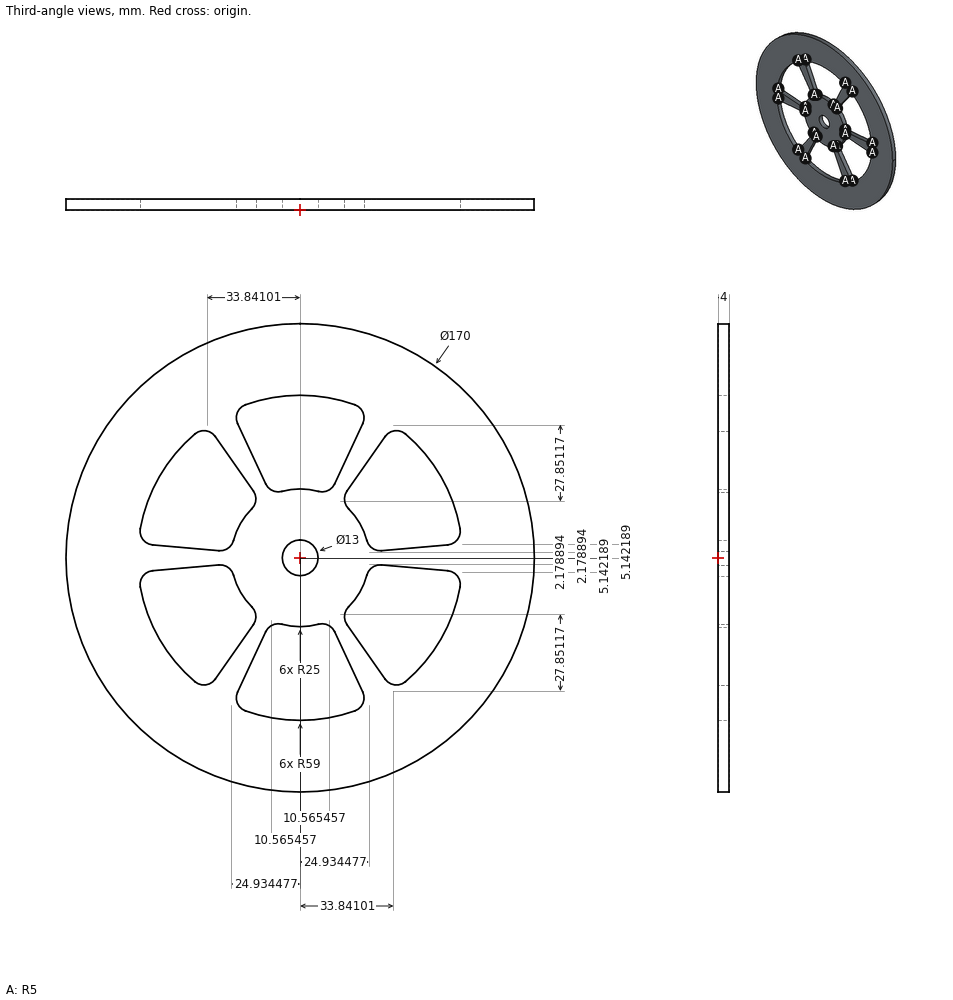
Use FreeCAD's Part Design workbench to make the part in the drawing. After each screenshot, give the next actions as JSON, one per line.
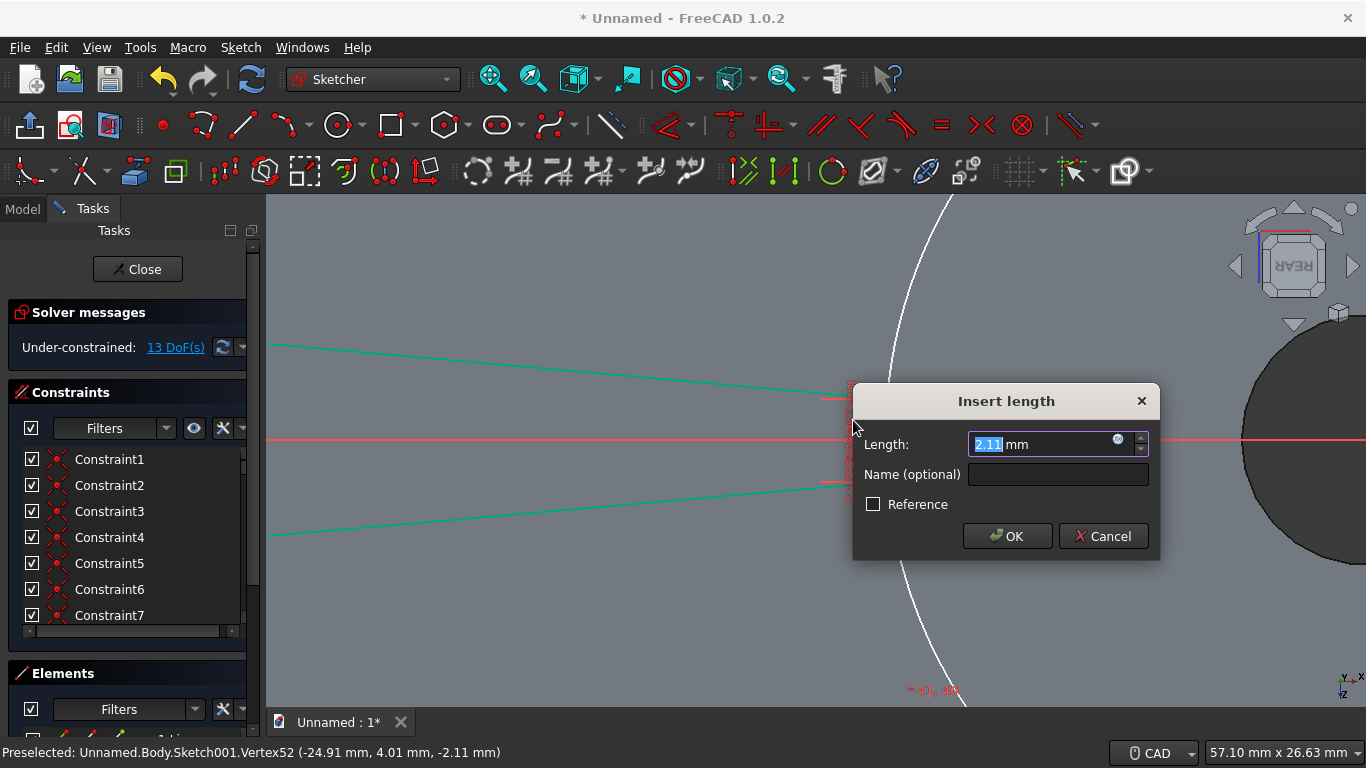
{"action": "type", "text": "2.178894"}
{"action": "key", "text": "Return"}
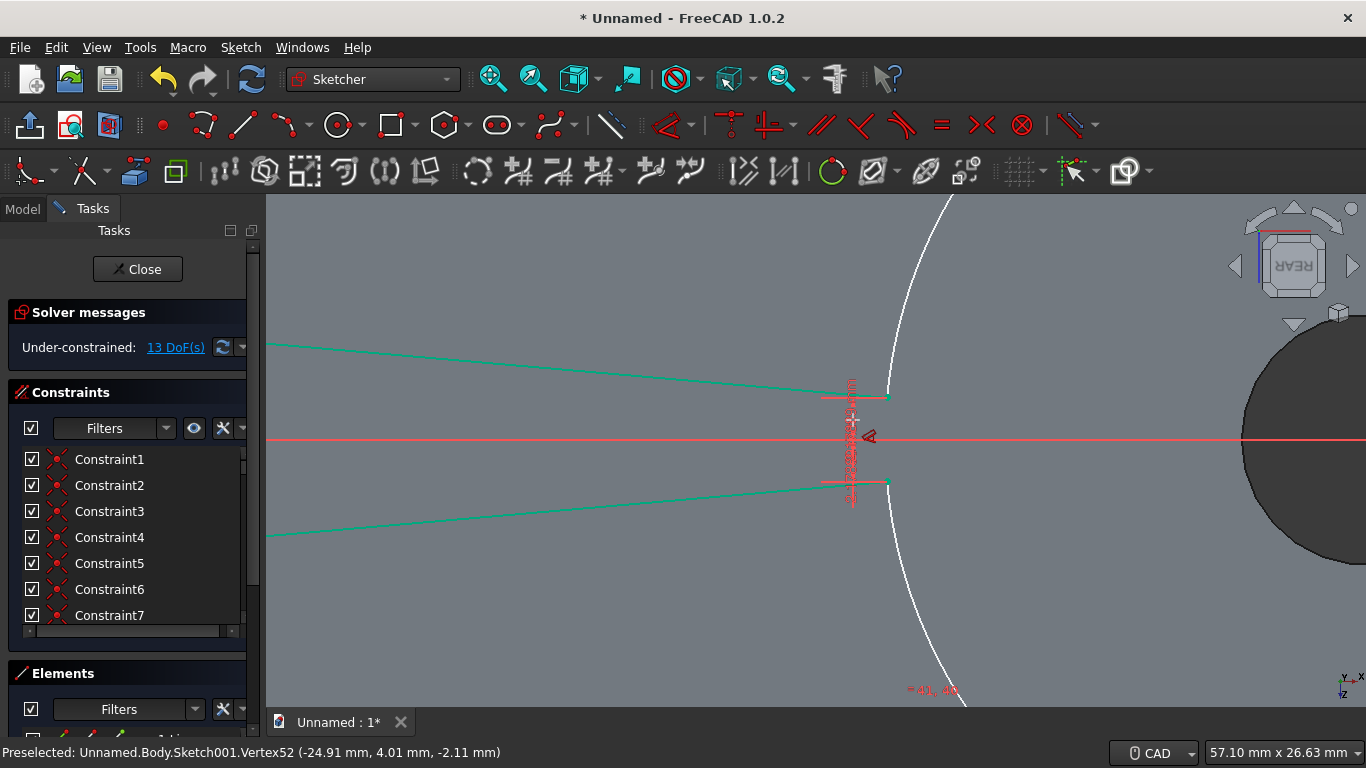
{"action": "scroll", "coordinate": [651, 452], "scroll_direction": "down", "scroll_amount": 10}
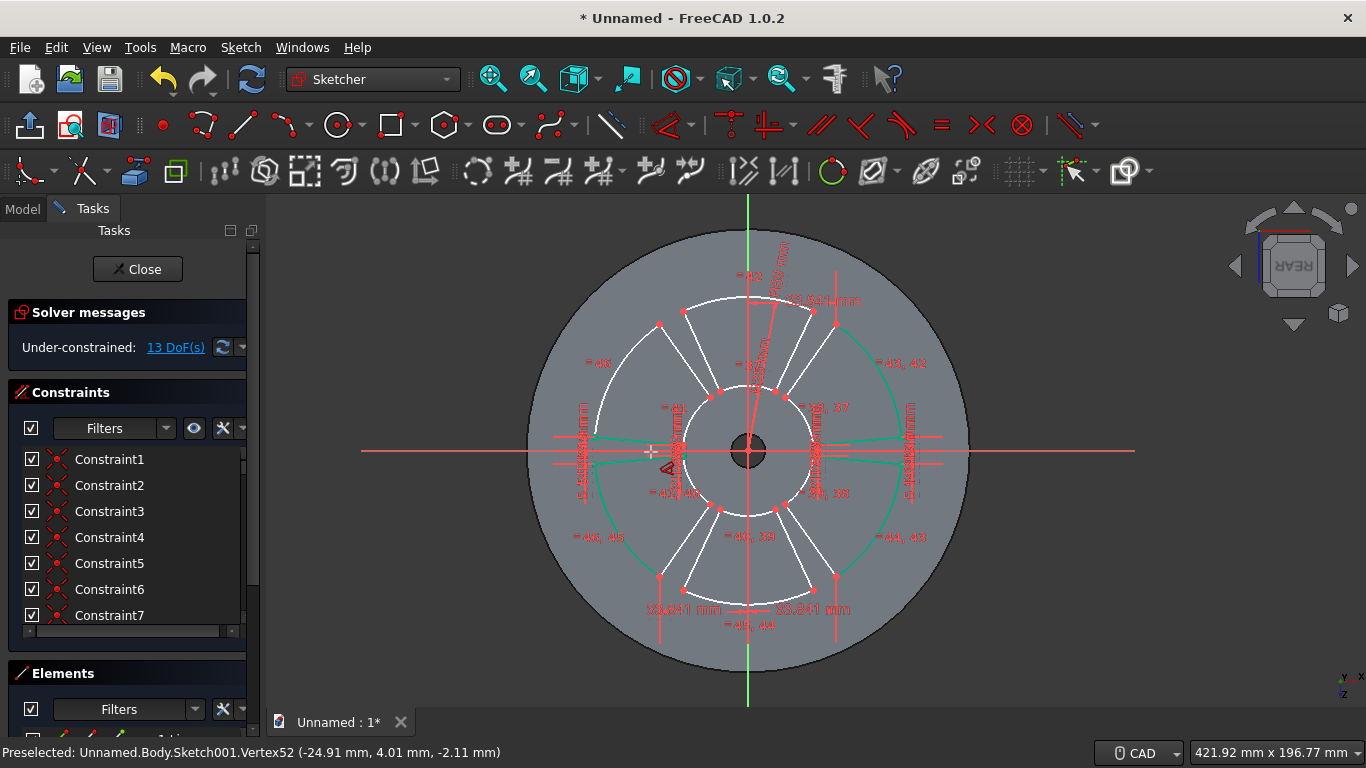
{"action": "left_click", "coordinate": [660, 325]}
{"action": "left_click", "coordinate": [684, 291]}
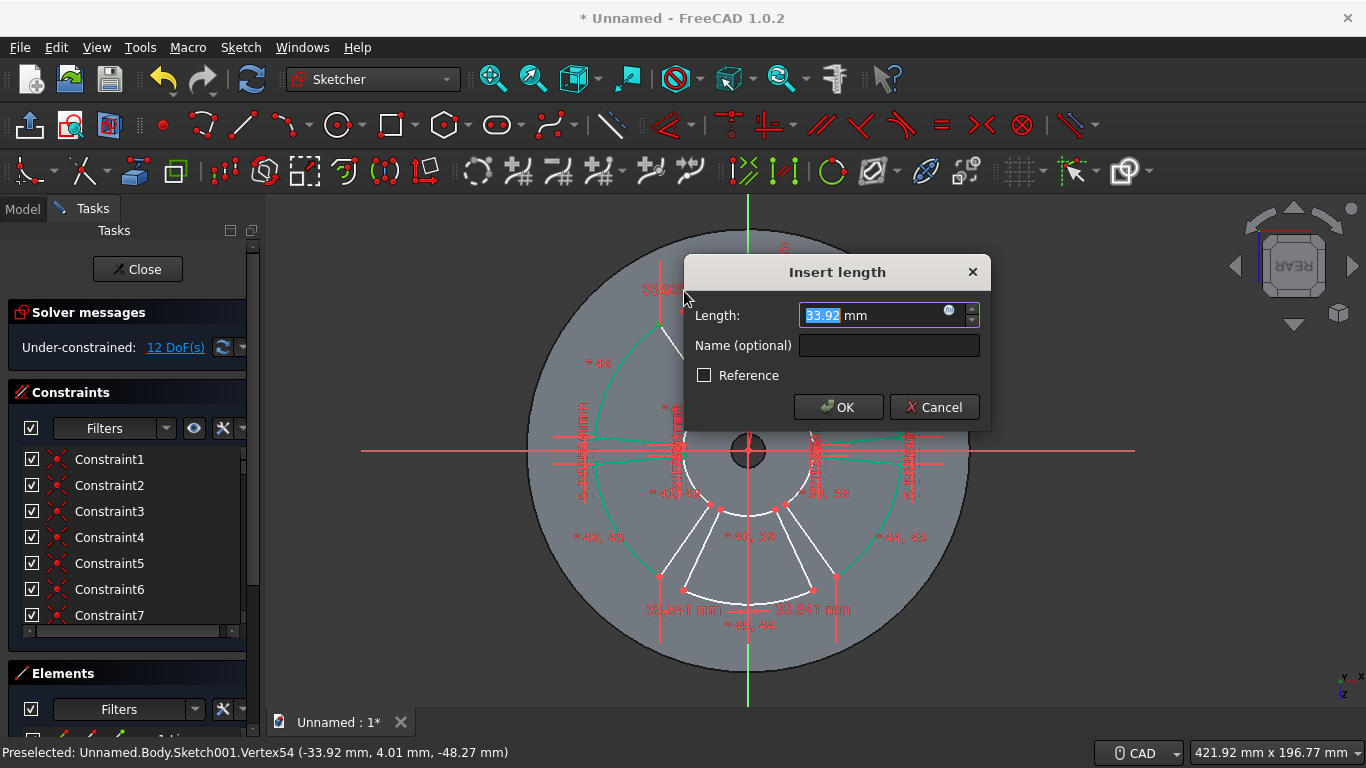
{"action": "type", "text": "33.84101"}
{"action": "key", "text": "Return"}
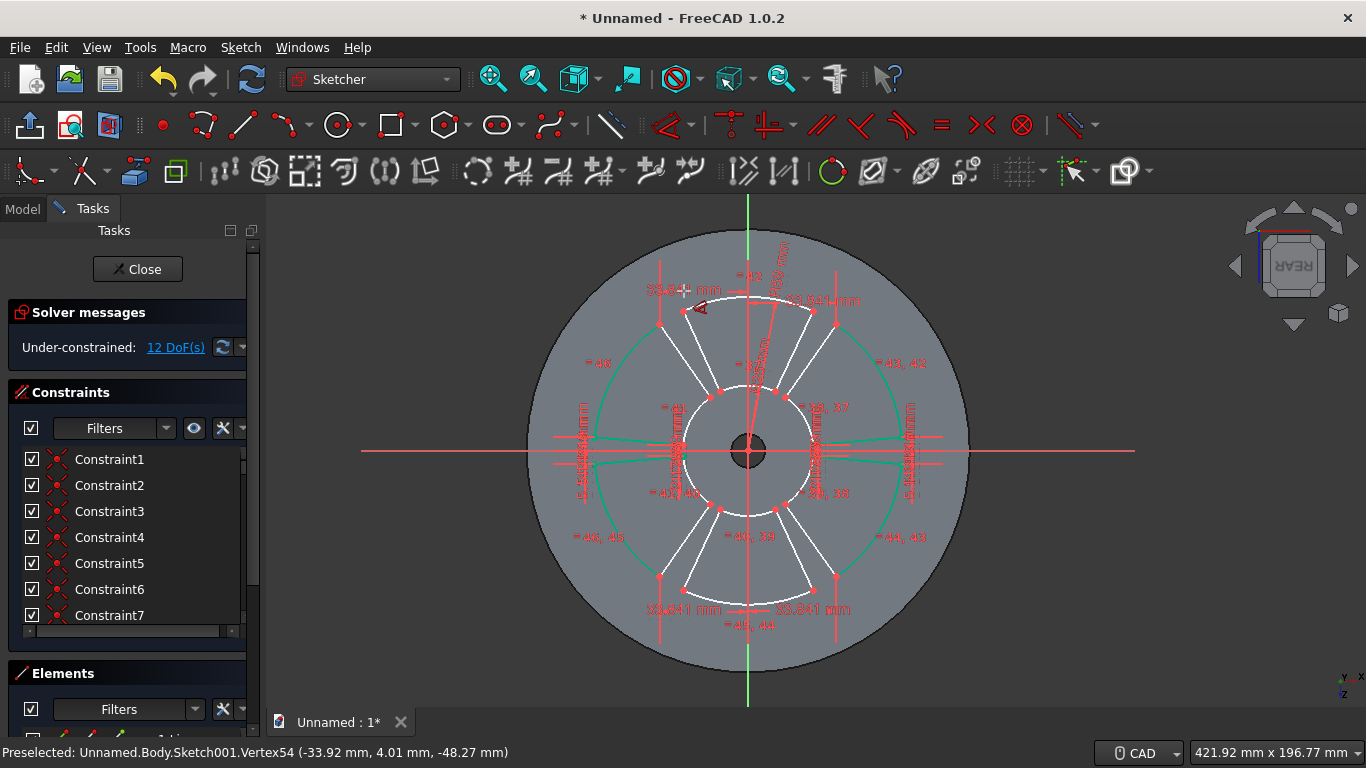
{"action": "left_click", "coordinate": [821, 347]}
{"action": "left_click", "coordinate": [870, 336]}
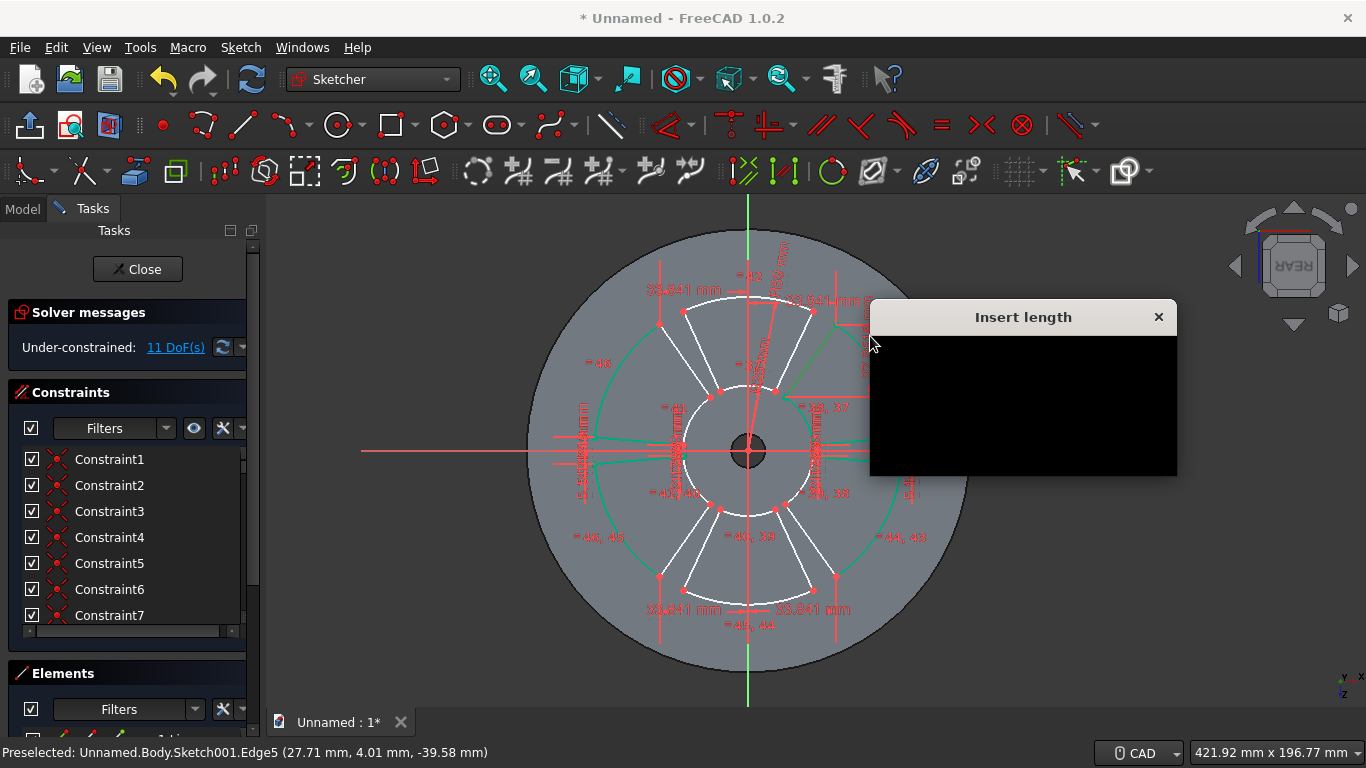
{"action": "type", "text": "27.85117"}
{"action": "key", "text": "Return"}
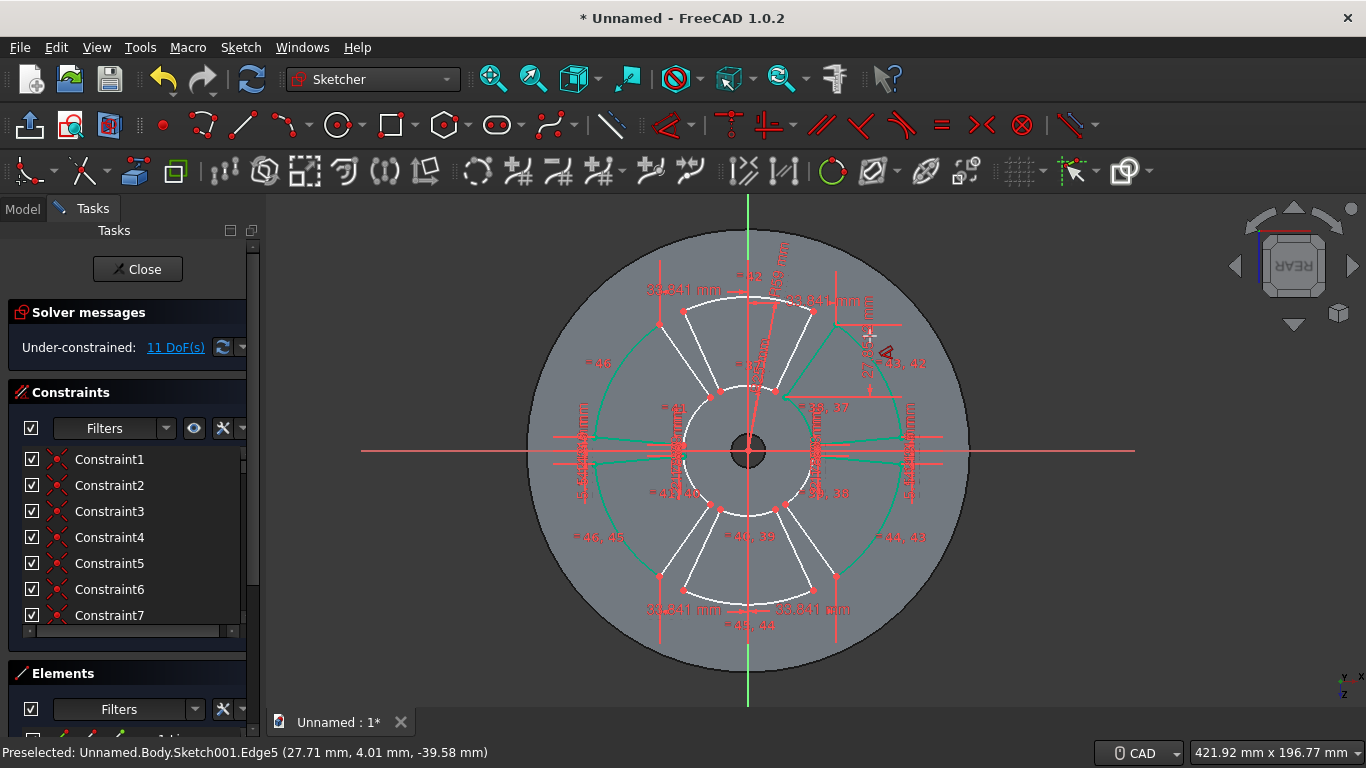
{"action": "left_click", "coordinate": [801, 526]}
{"action": "left_click", "coordinate": [870, 515]}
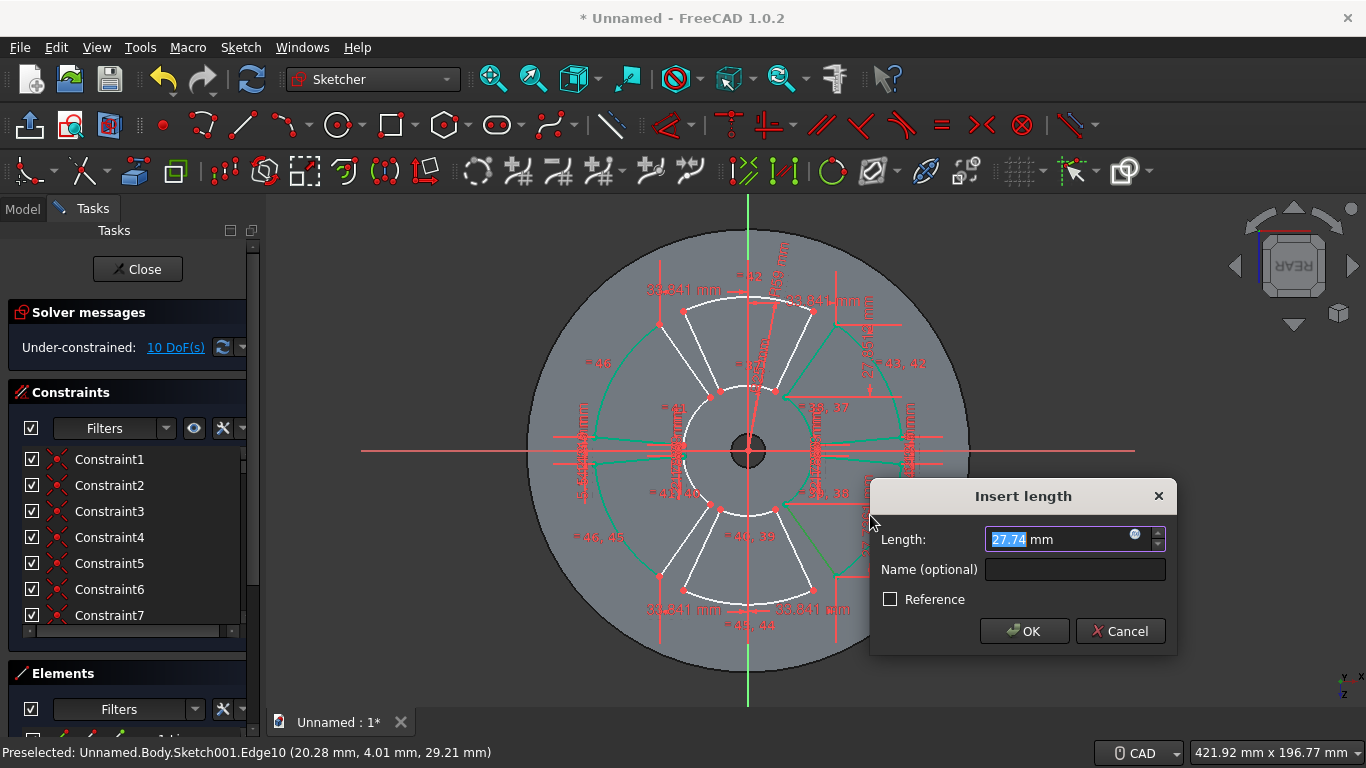
{"action": "type", "text": "27.85117"}
{"action": "key", "text": "Return"}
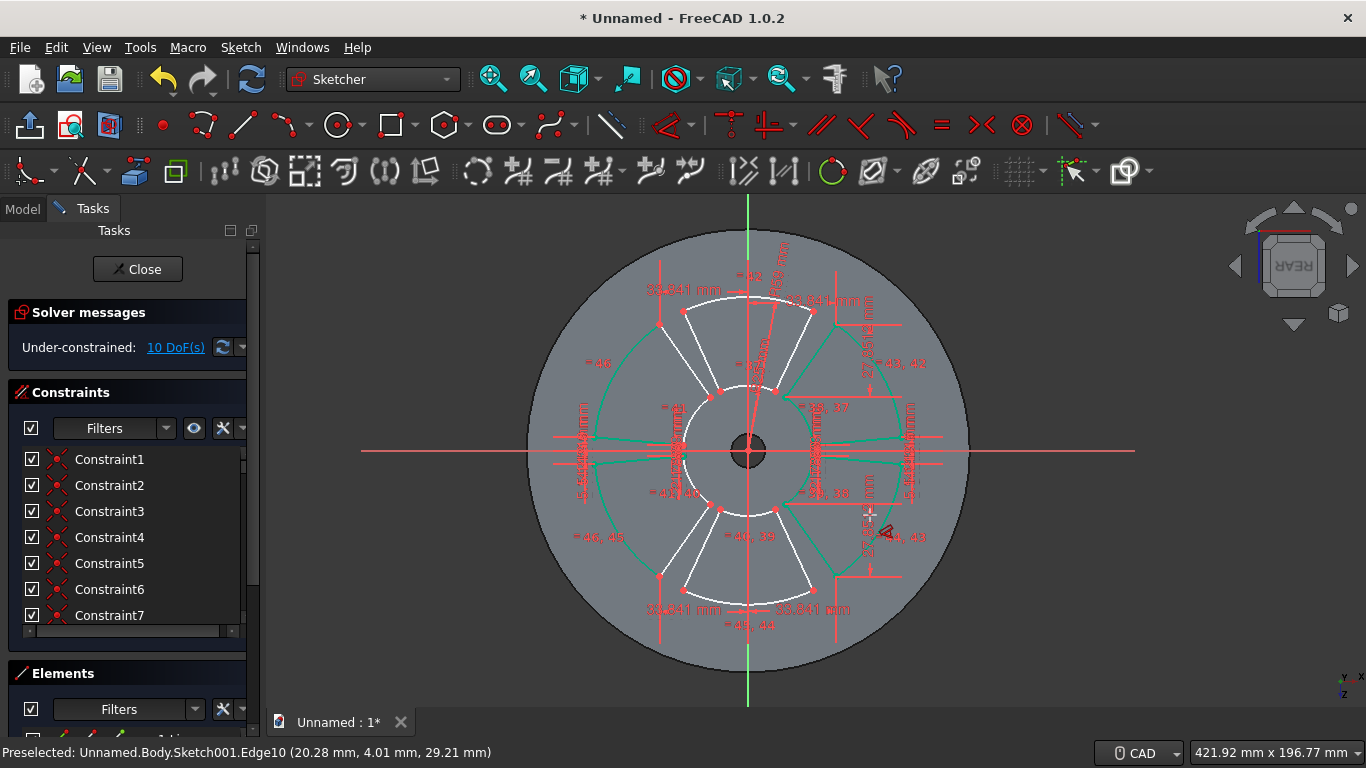
{"action": "left_click", "coordinate": [675, 555]}
{"action": "left_click", "coordinate": [626, 515]}